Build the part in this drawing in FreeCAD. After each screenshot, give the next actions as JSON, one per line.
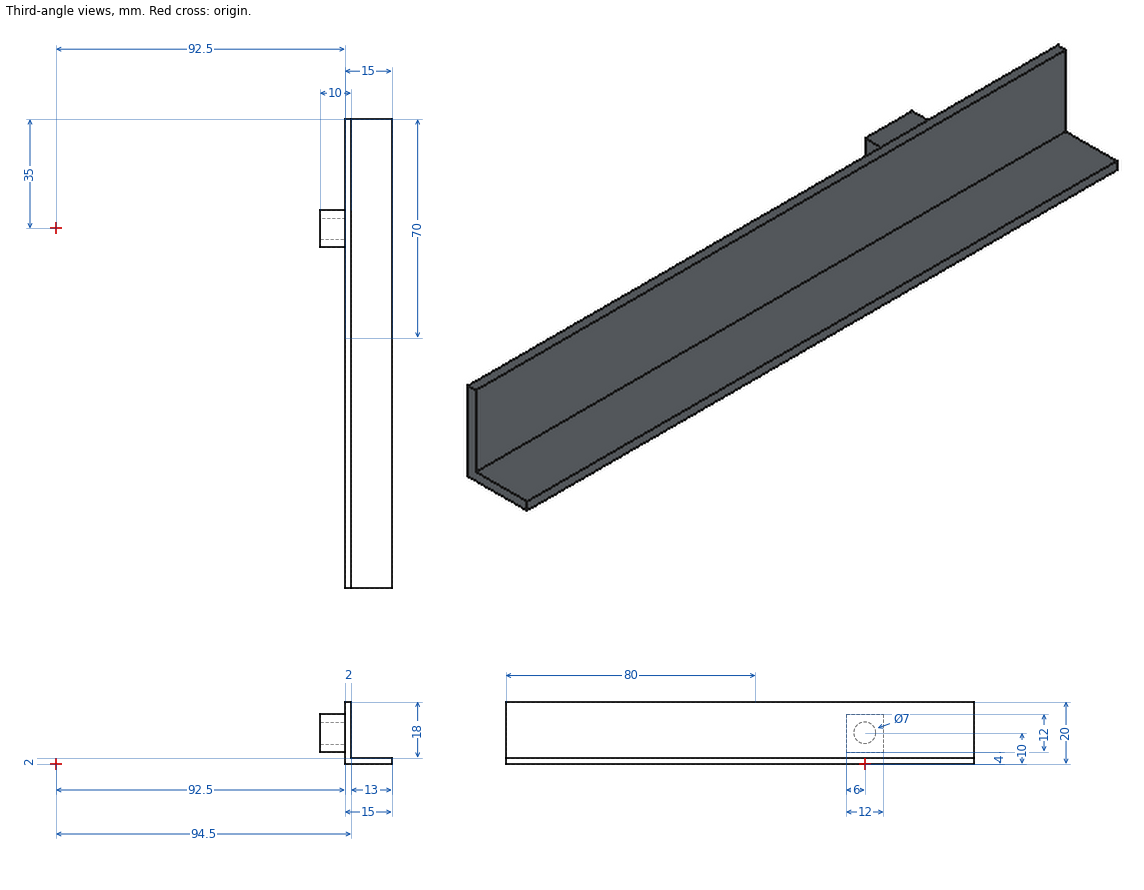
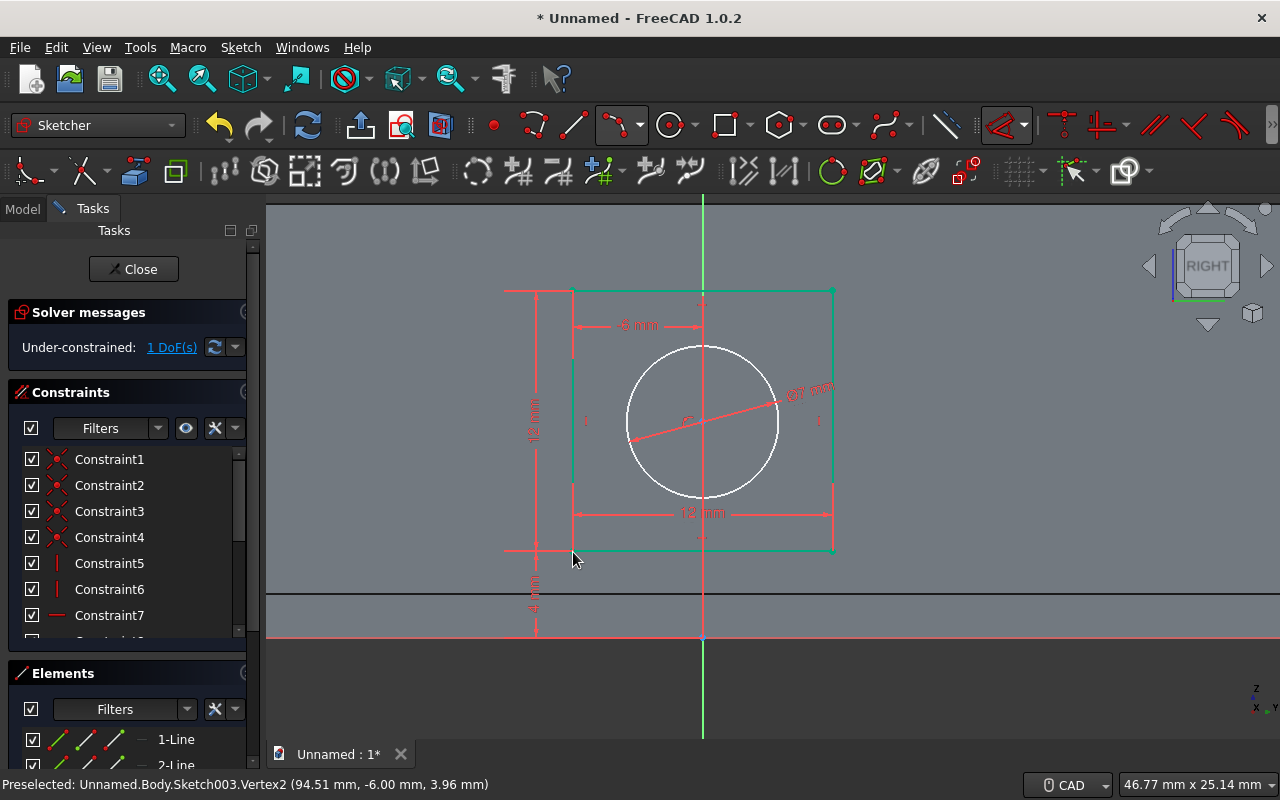
{"action": "left_click", "coordinate": [703, 422]}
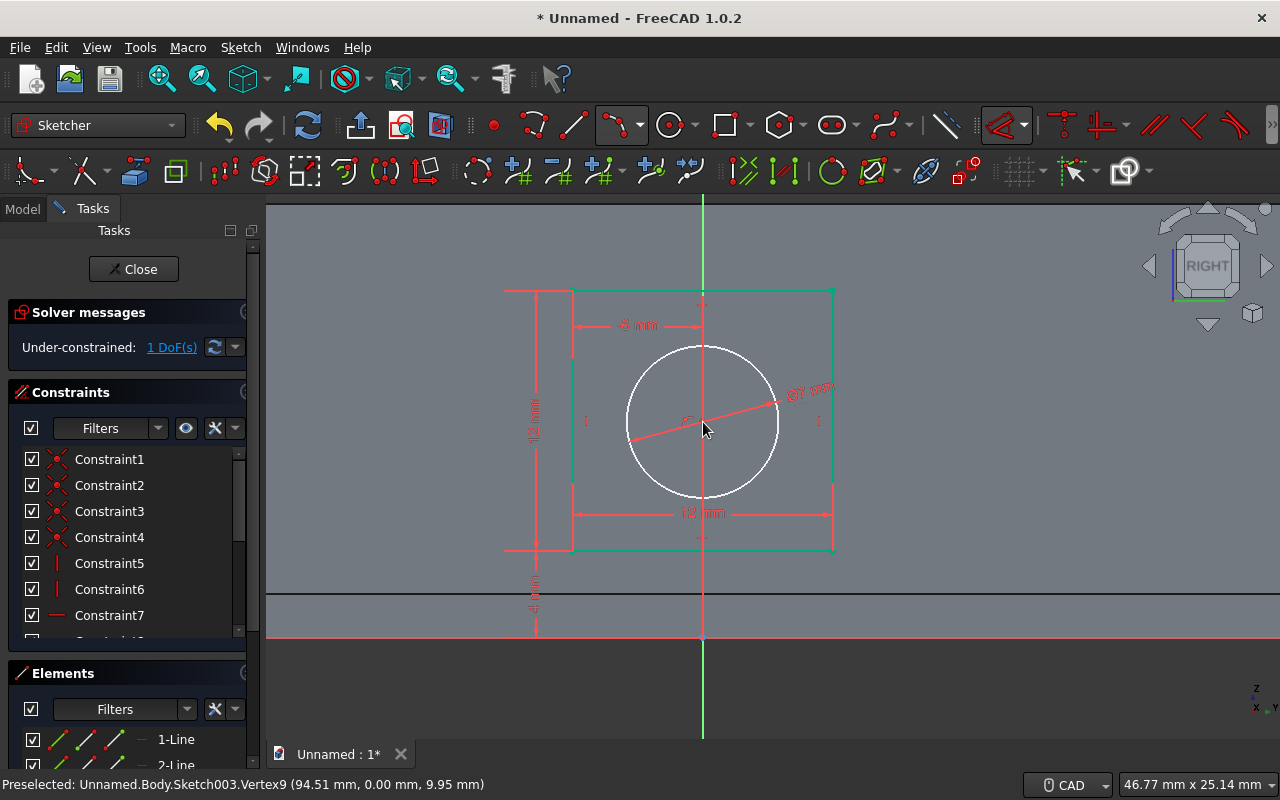
{"action": "key", "text": "i"}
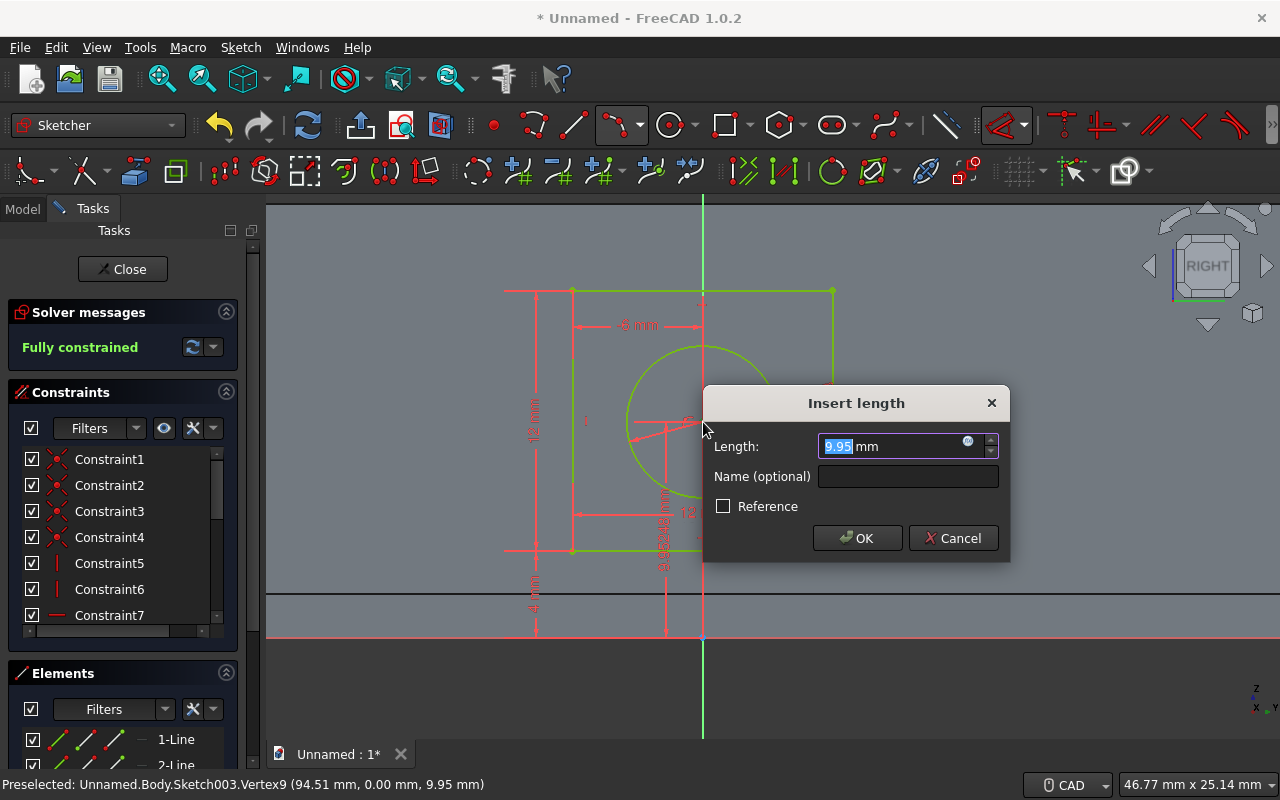
{"action": "type", "text": "10"}
{"action": "key", "text": "Return"}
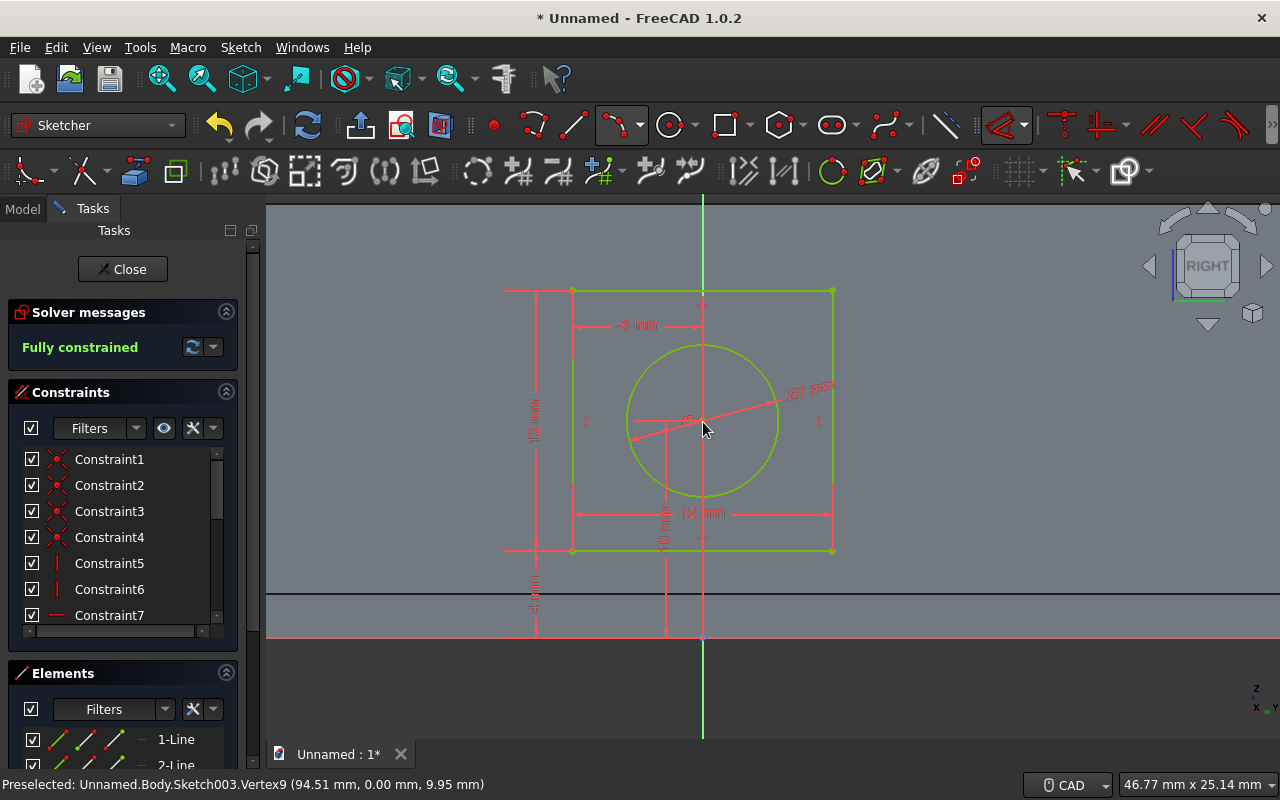
{"action": "left_click", "coordinate": [123, 269]}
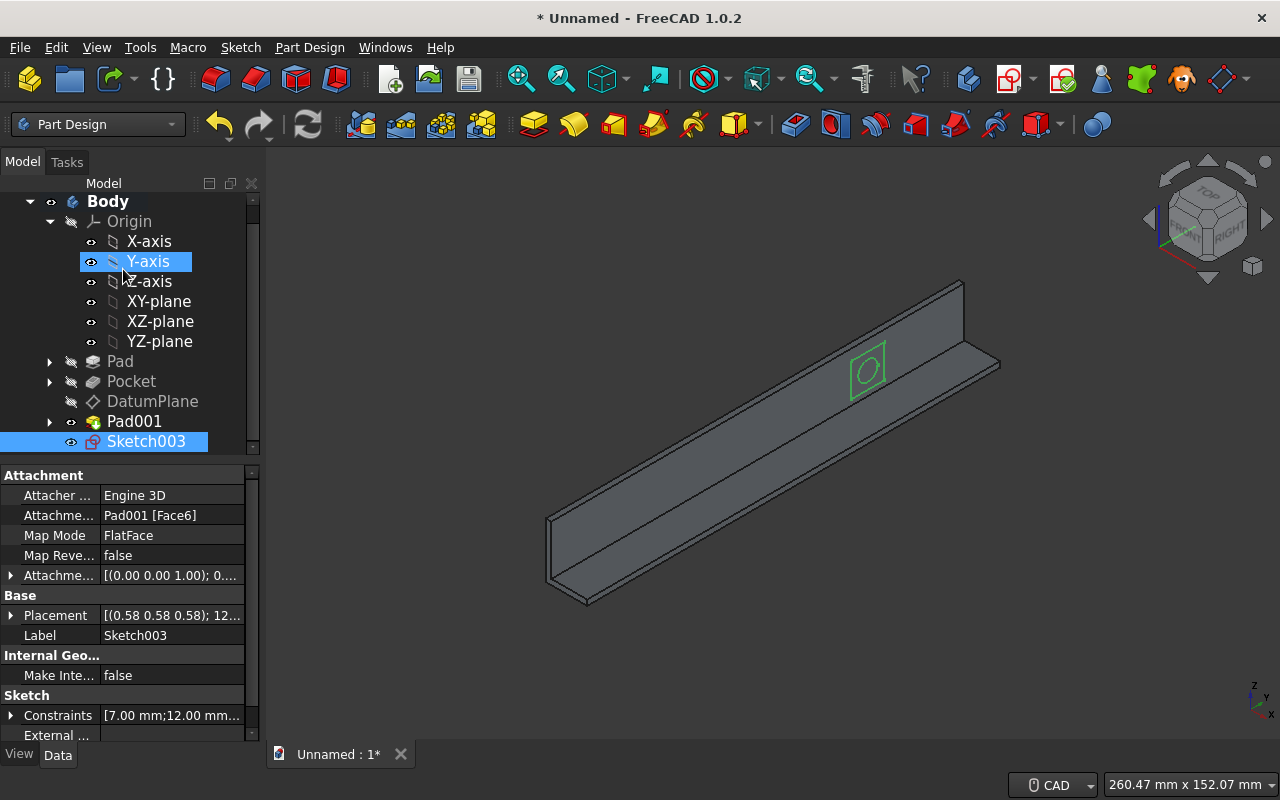
{"action": "left_click", "coordinate": [534, 124]}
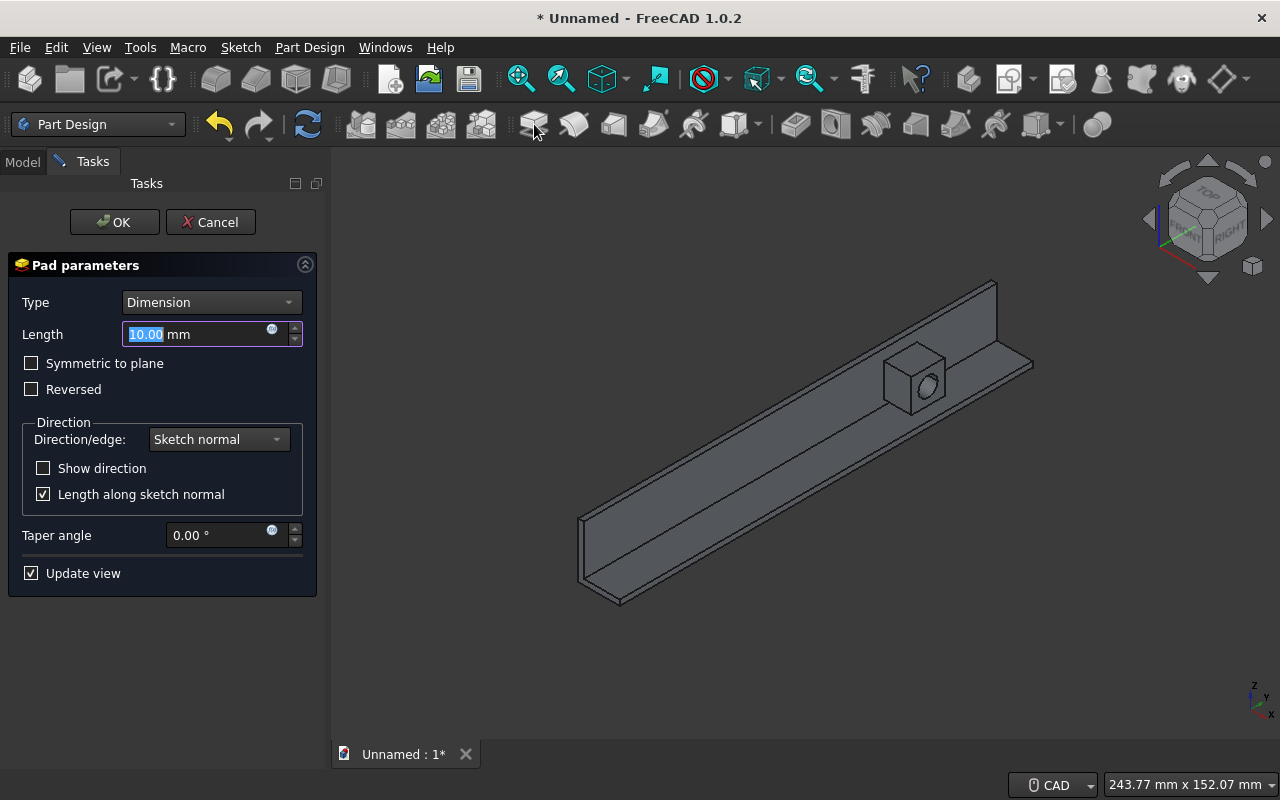
{"action": "type", "text": "10"}
{"action": "key", "text": "Tab"}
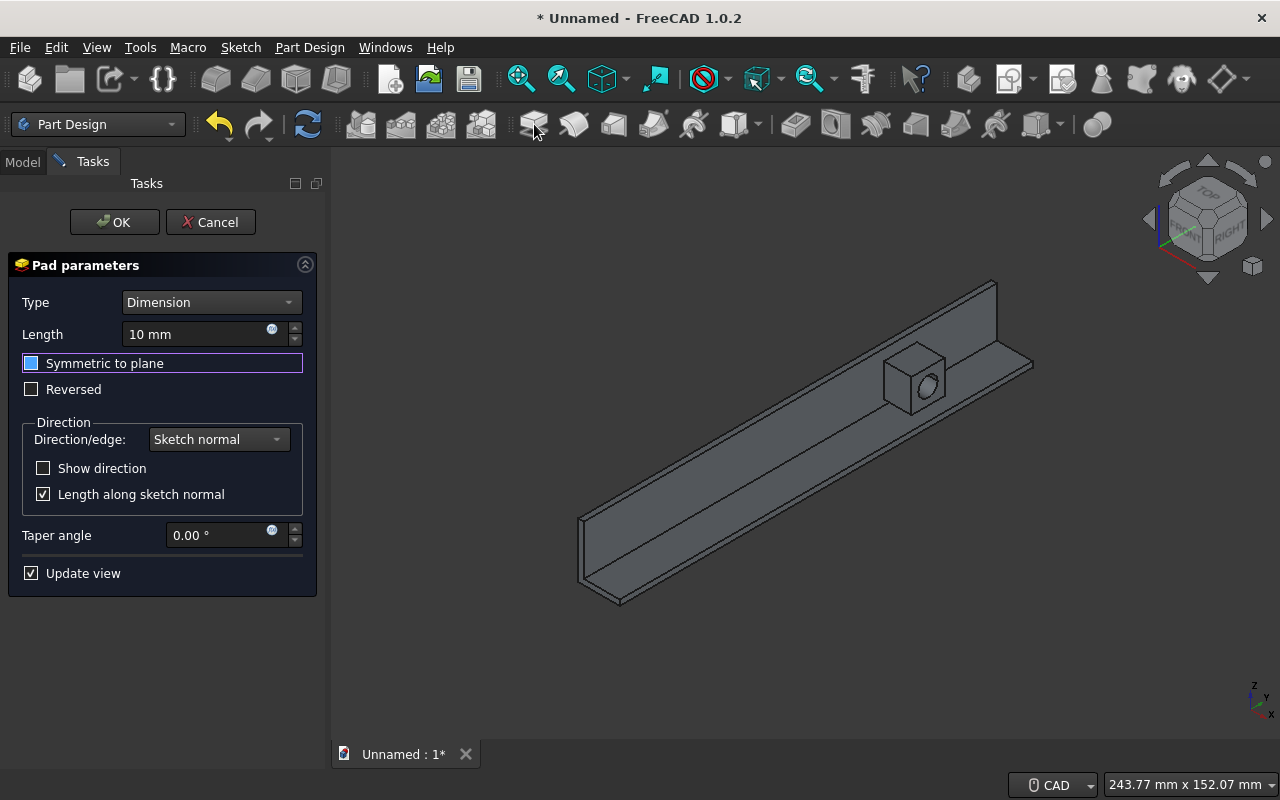
{"action": "left_click", "coordinate": [30, 389]}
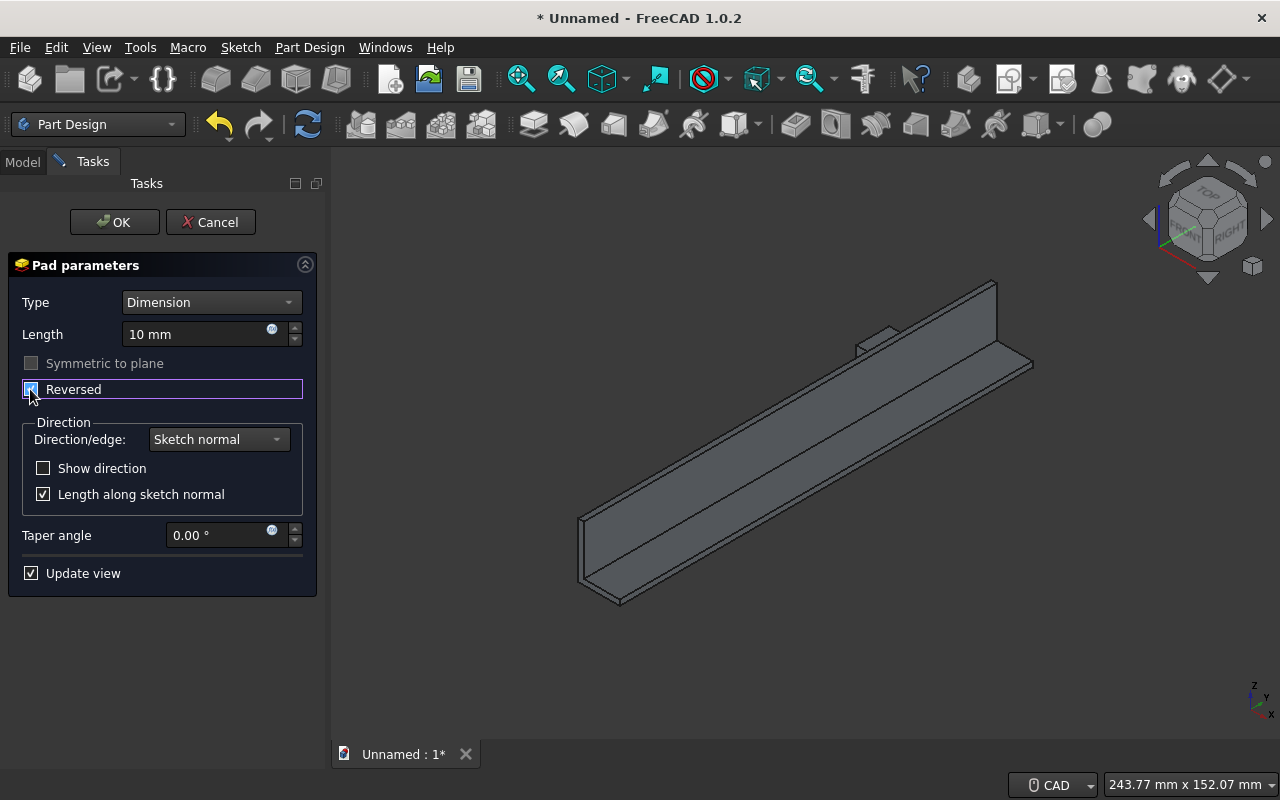
{"action": "left_click", "coordinate": [115, 222]}